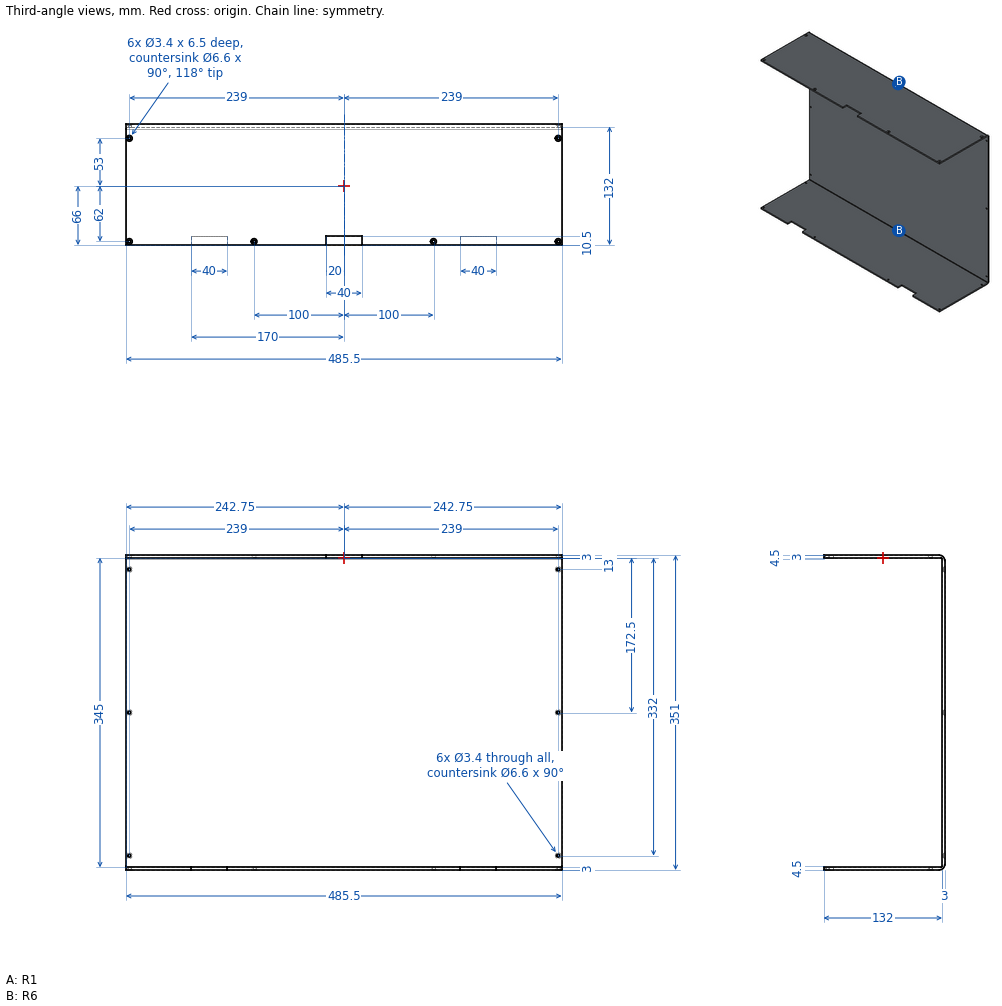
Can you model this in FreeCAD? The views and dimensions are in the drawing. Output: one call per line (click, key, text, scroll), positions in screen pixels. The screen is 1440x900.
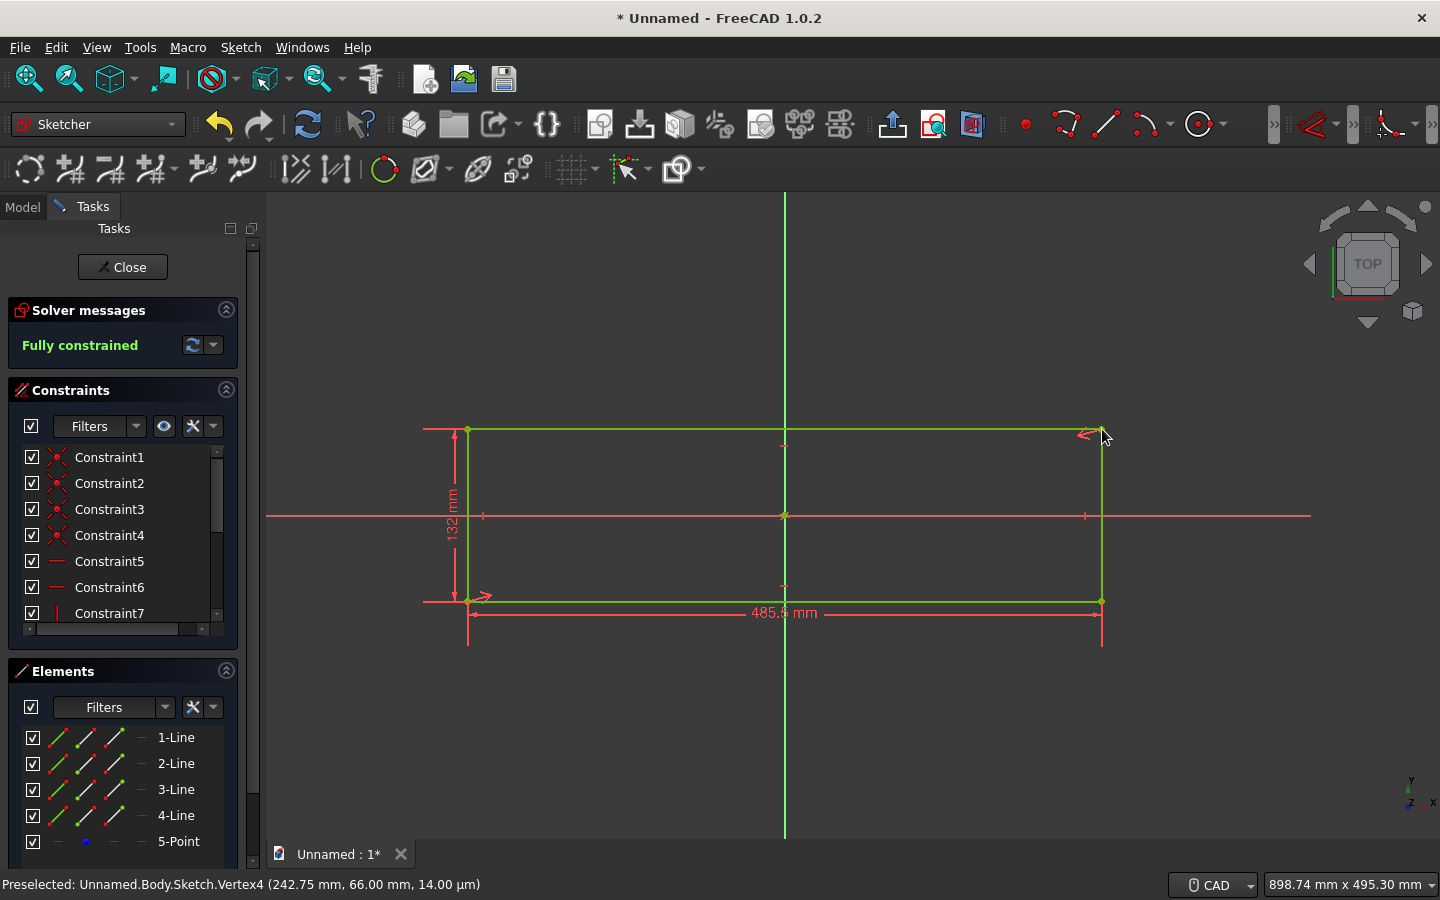
click(123, 267)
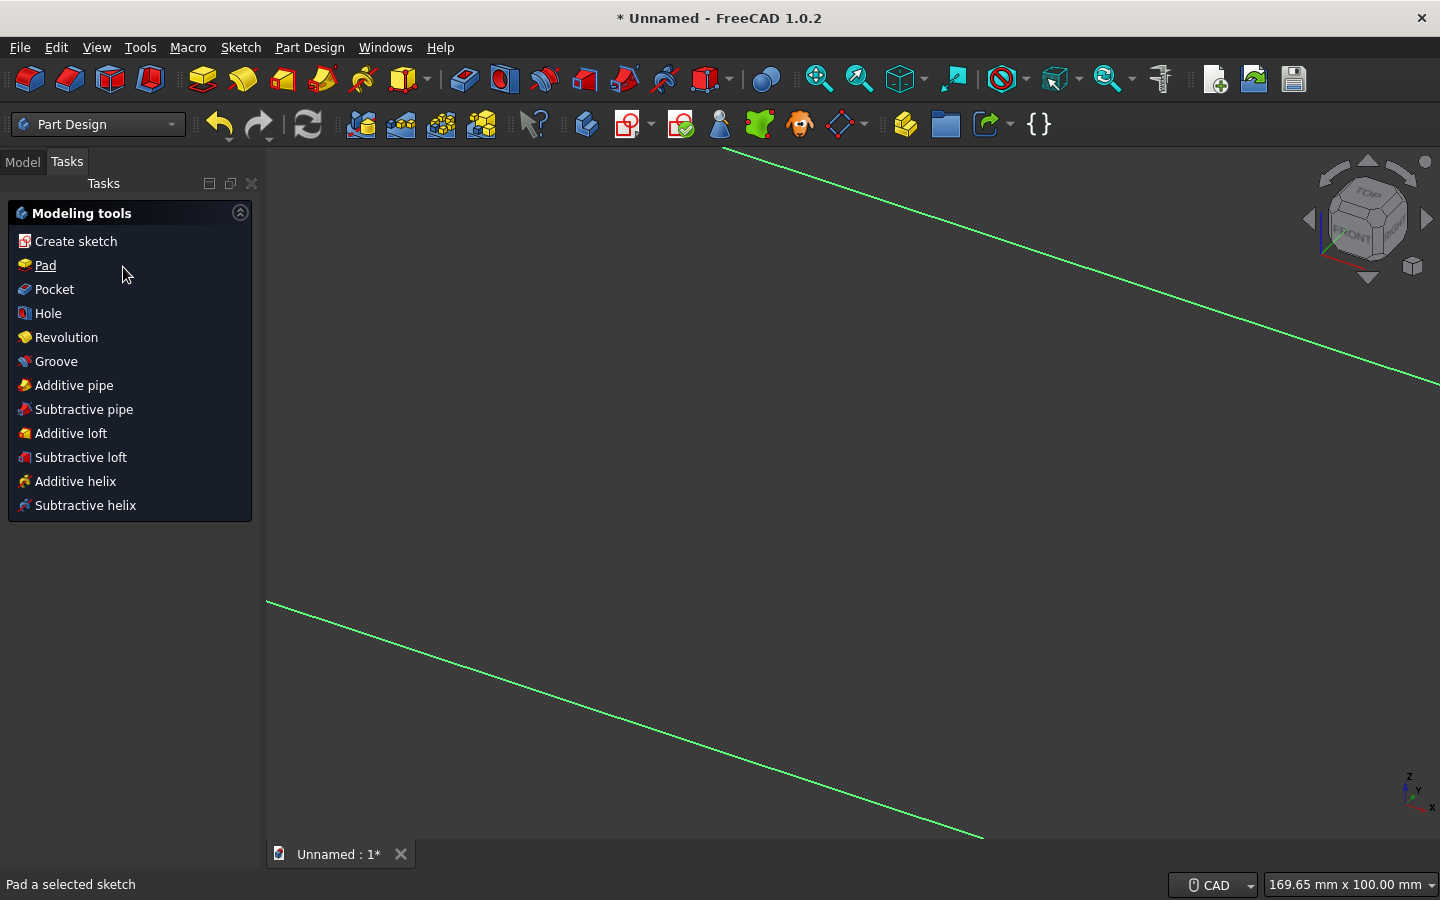
click(204, 80)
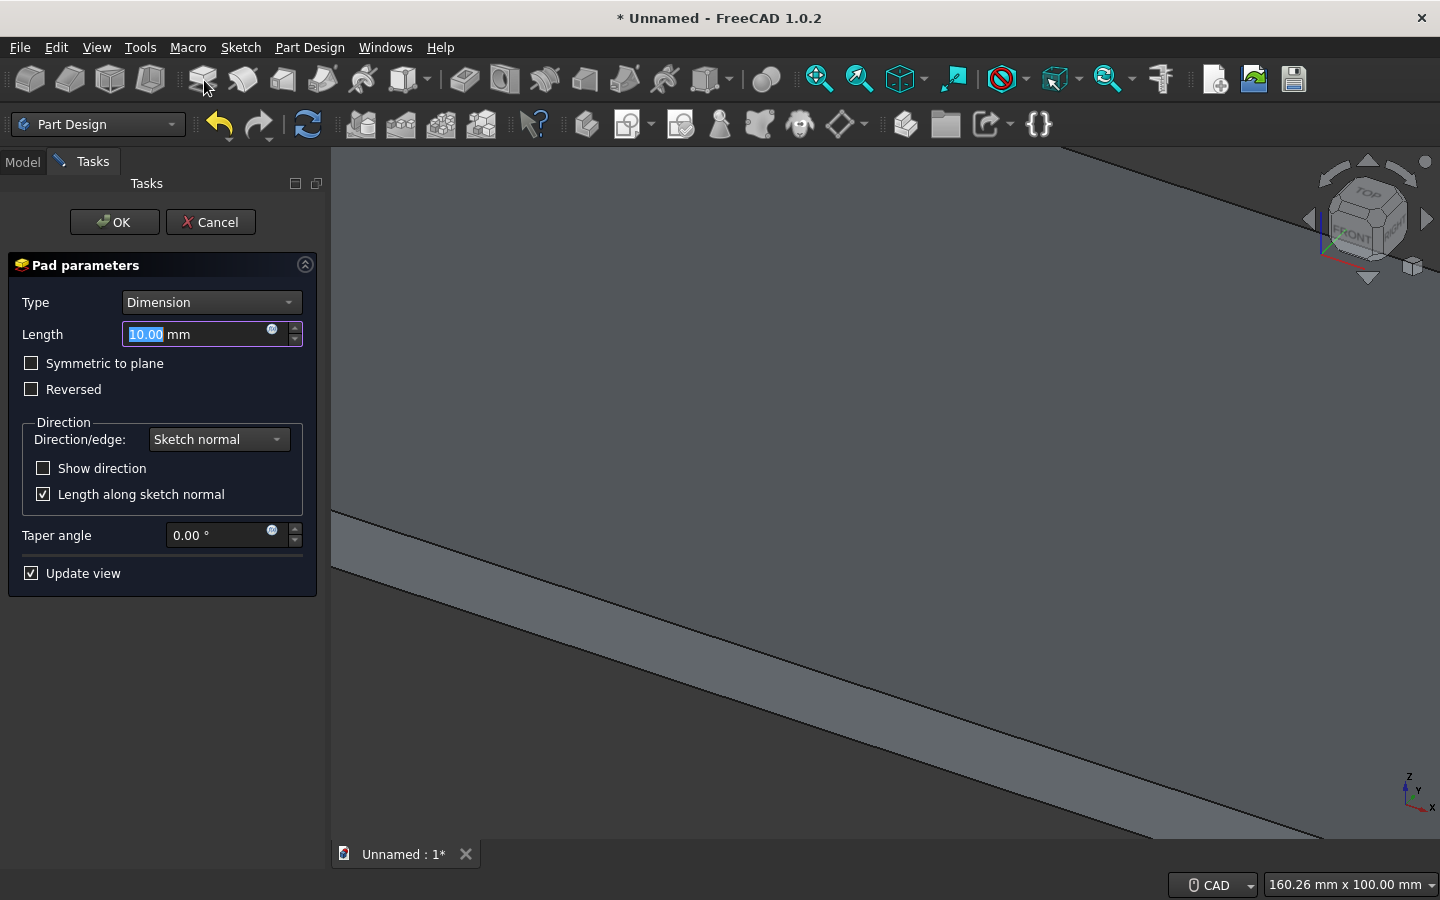
text(3)
key(Tab)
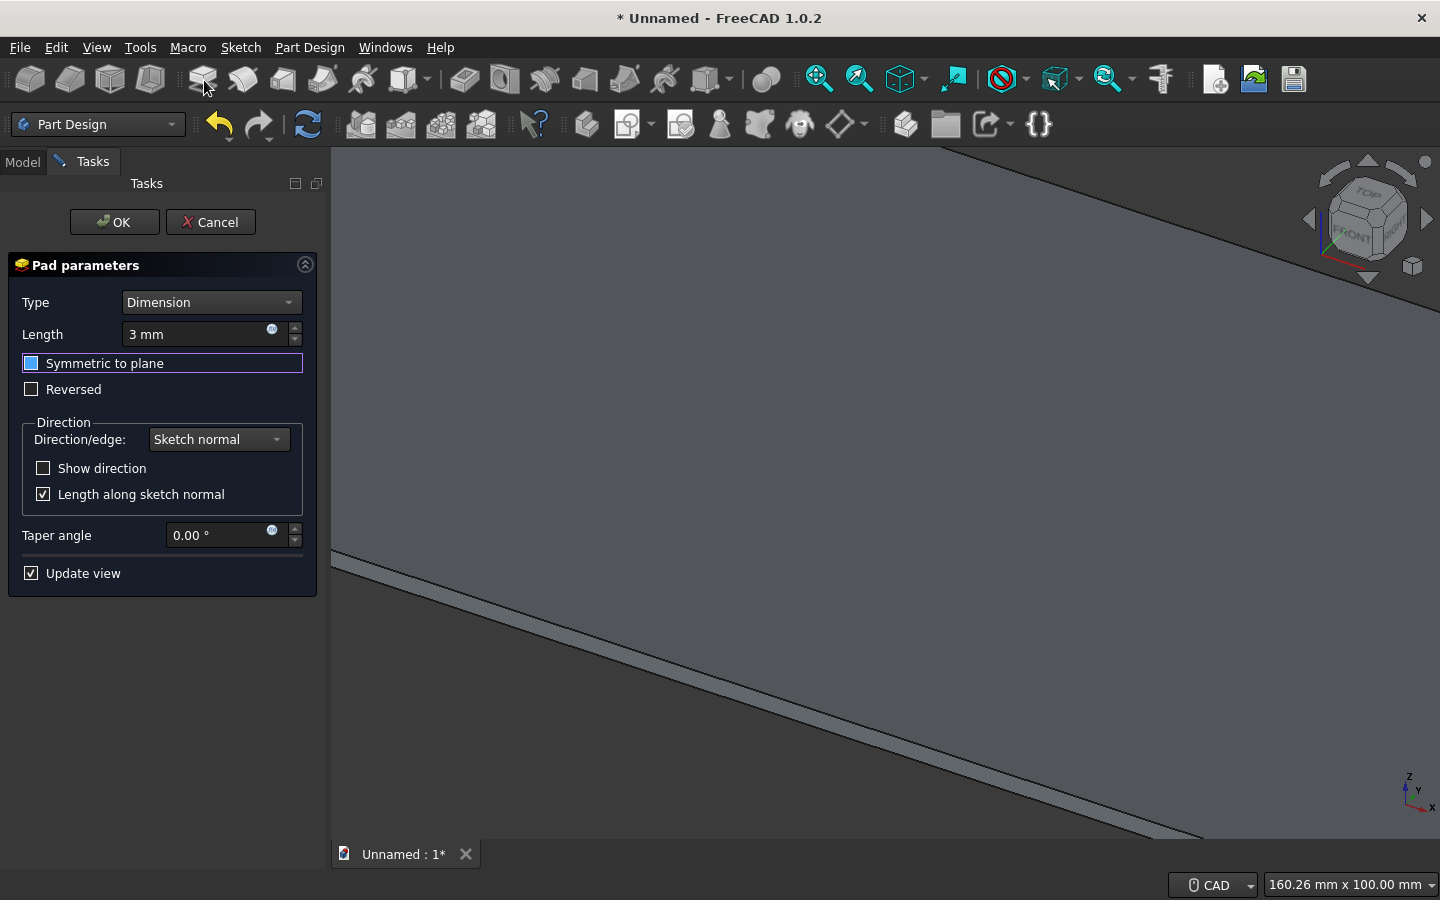
click(115, 222)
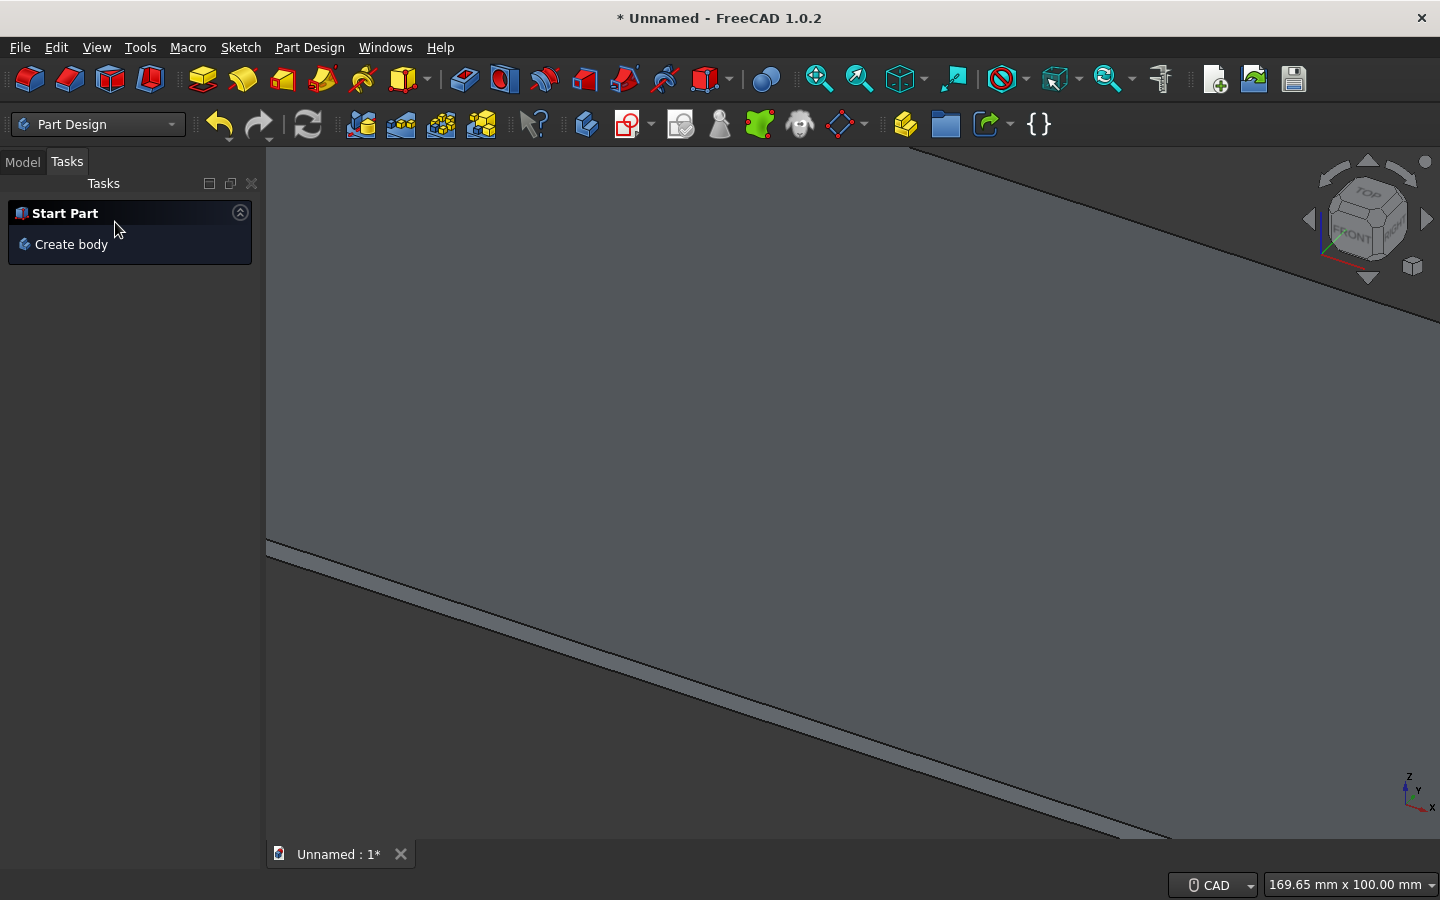
click(820, 80)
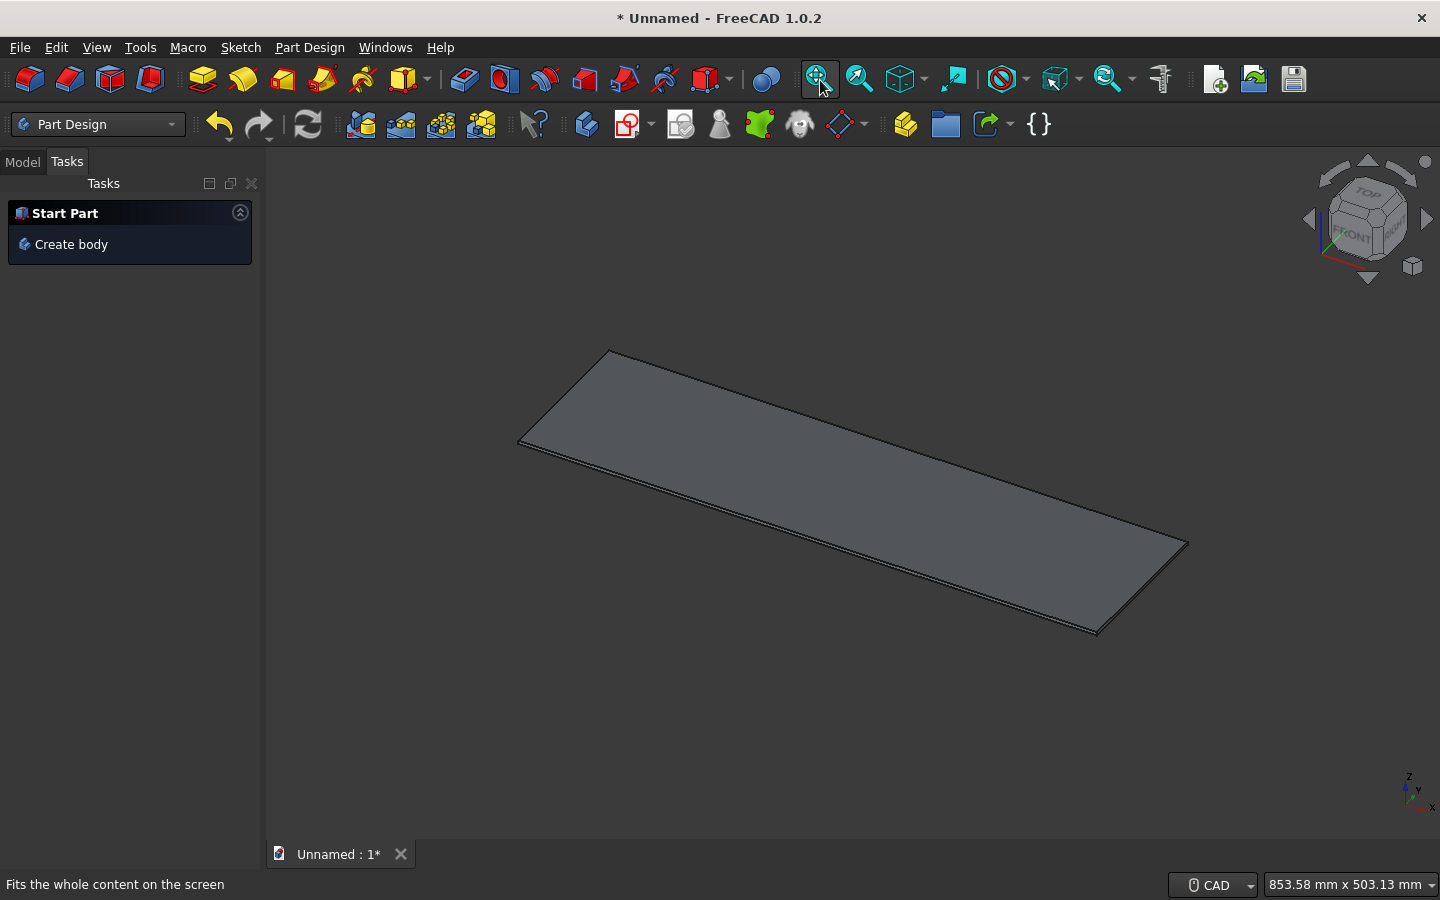
key(4)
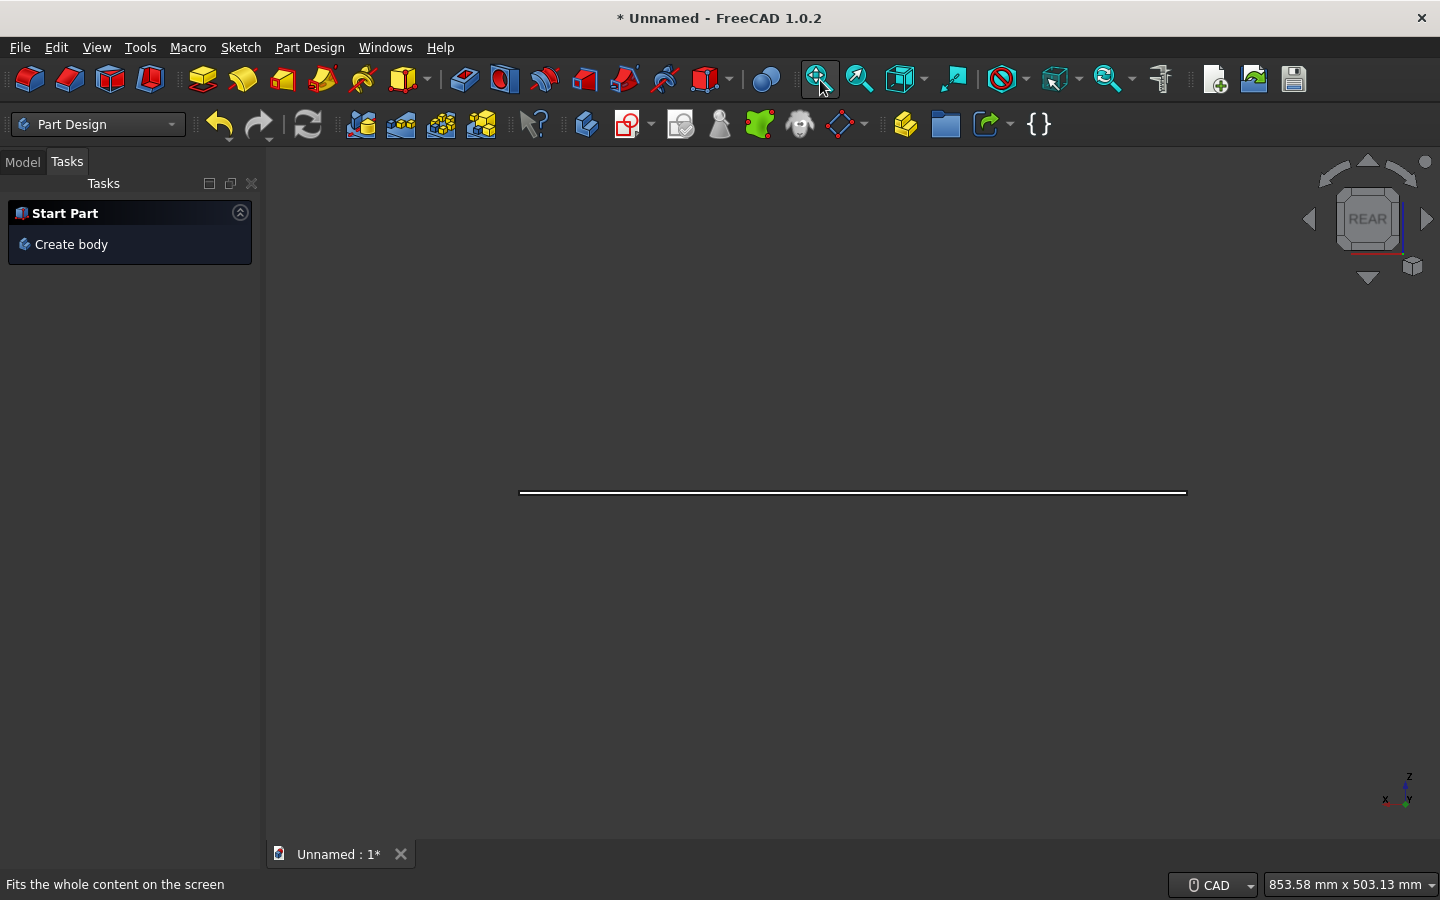
scroll(567, 492, up, 9)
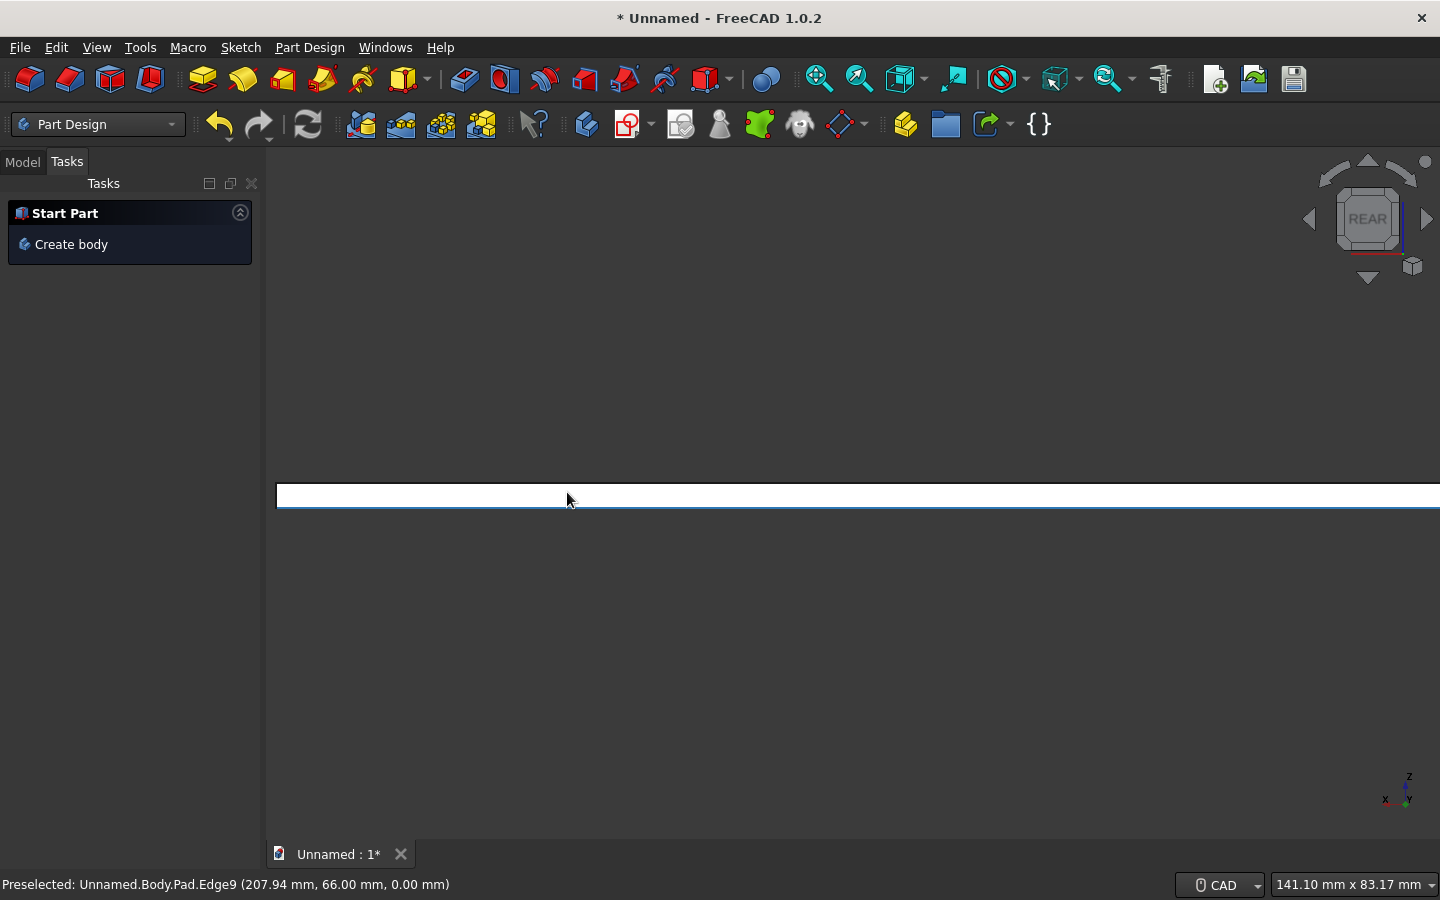
click(565, 495)